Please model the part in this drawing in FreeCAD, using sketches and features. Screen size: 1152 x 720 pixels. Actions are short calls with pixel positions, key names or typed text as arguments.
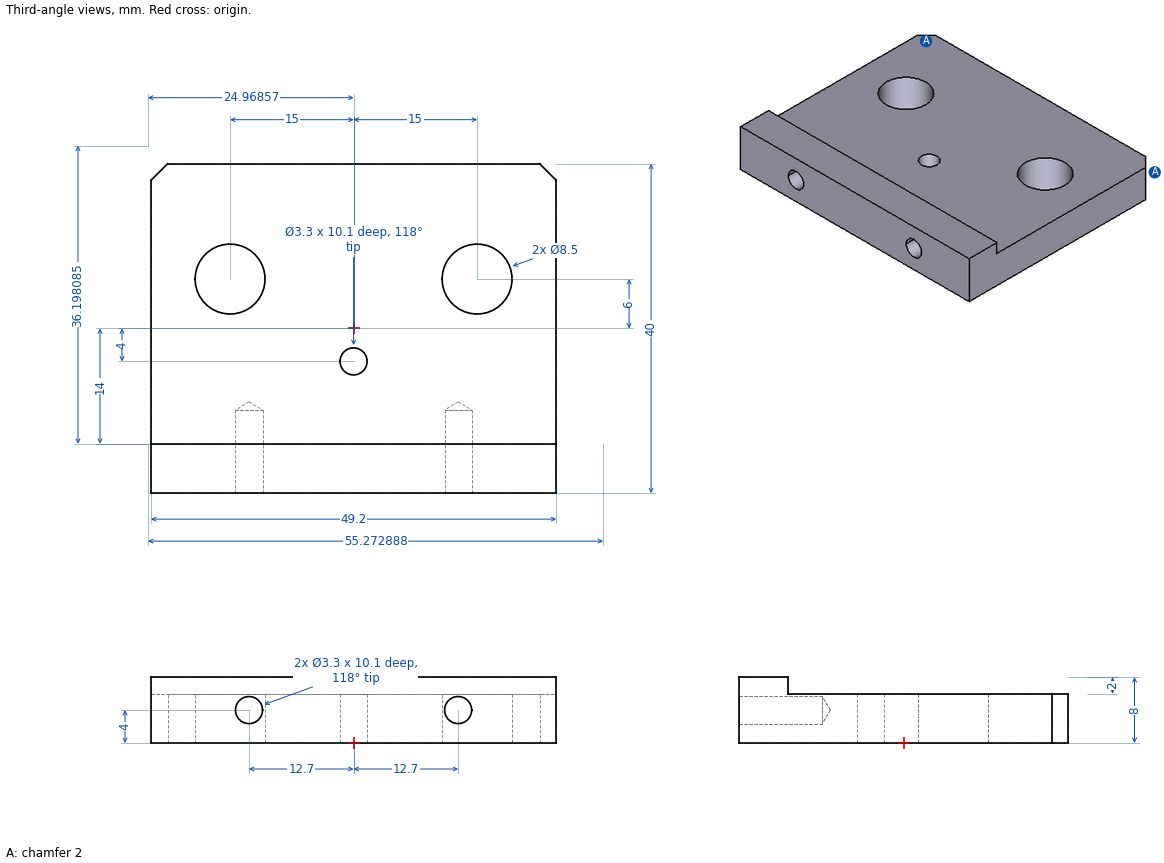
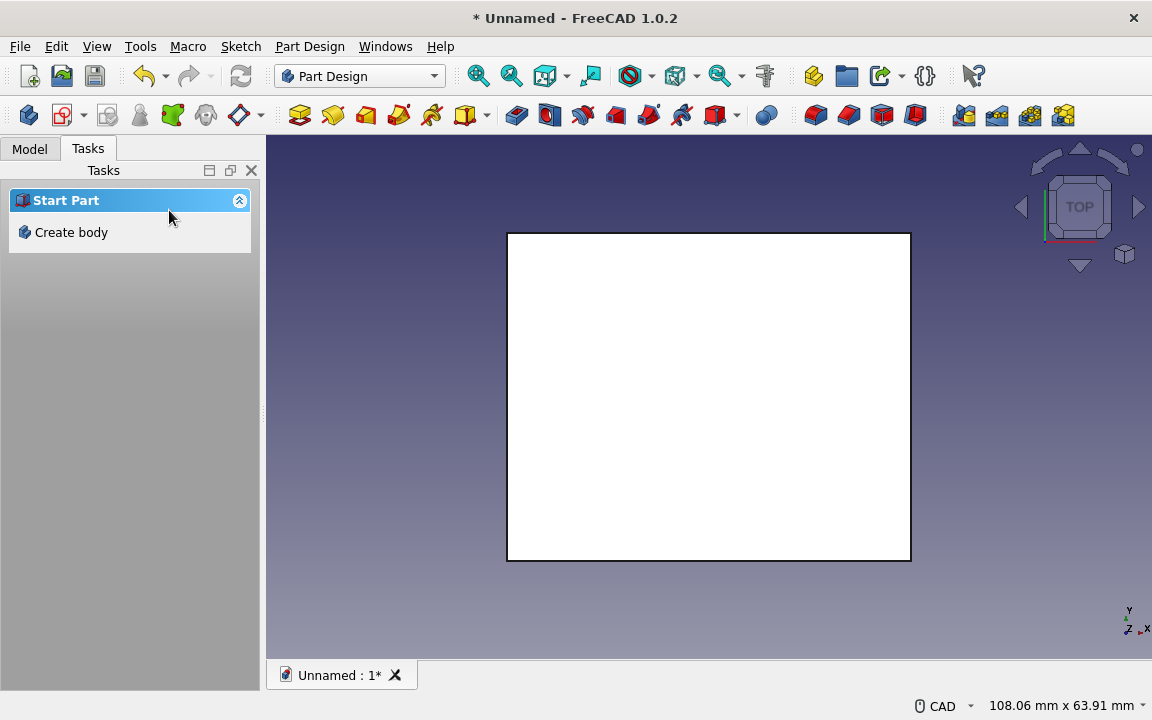
key(1)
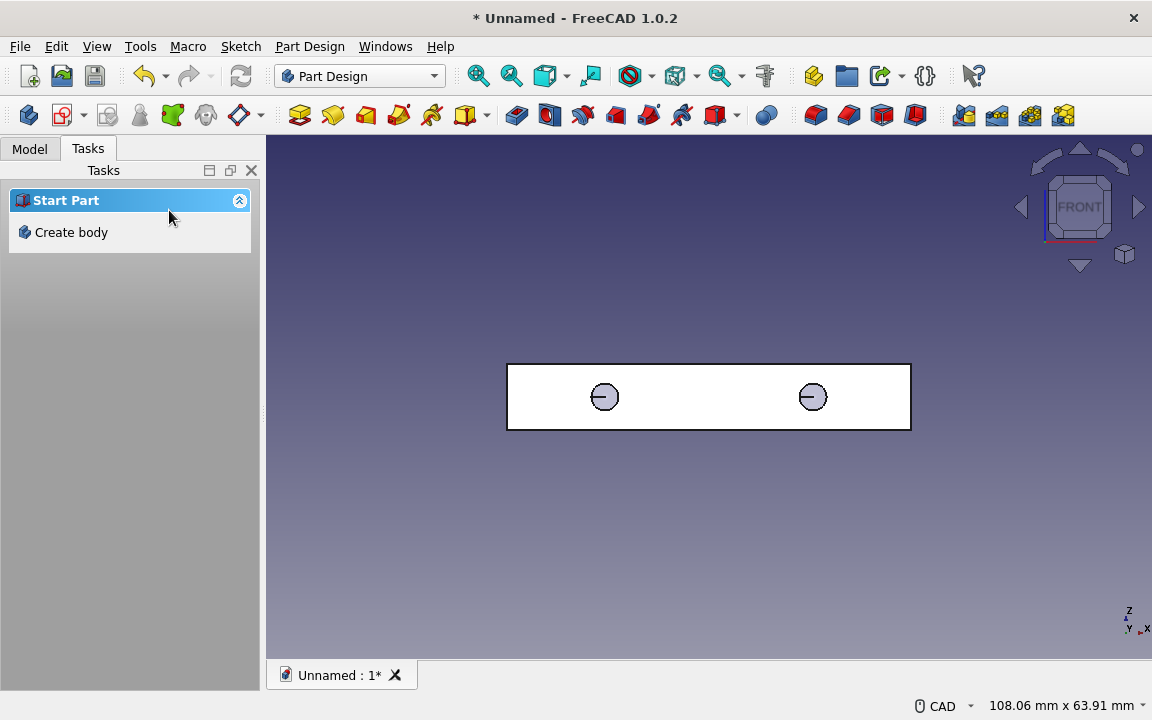
key(3)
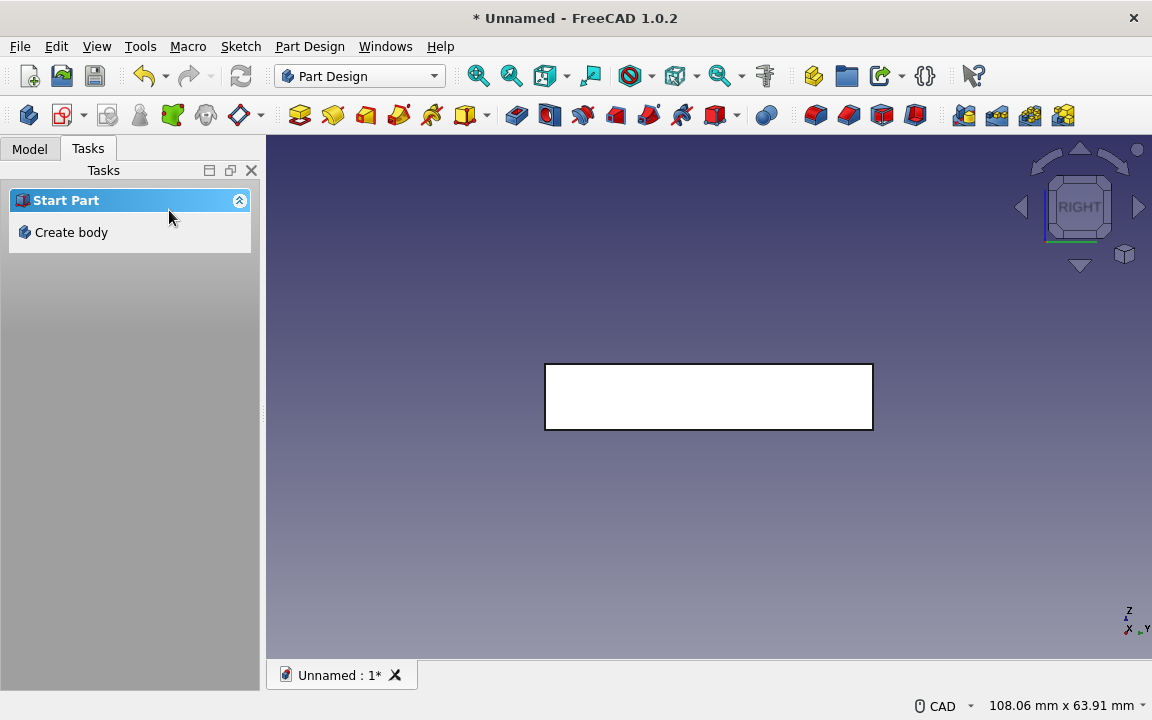
click(479, 76)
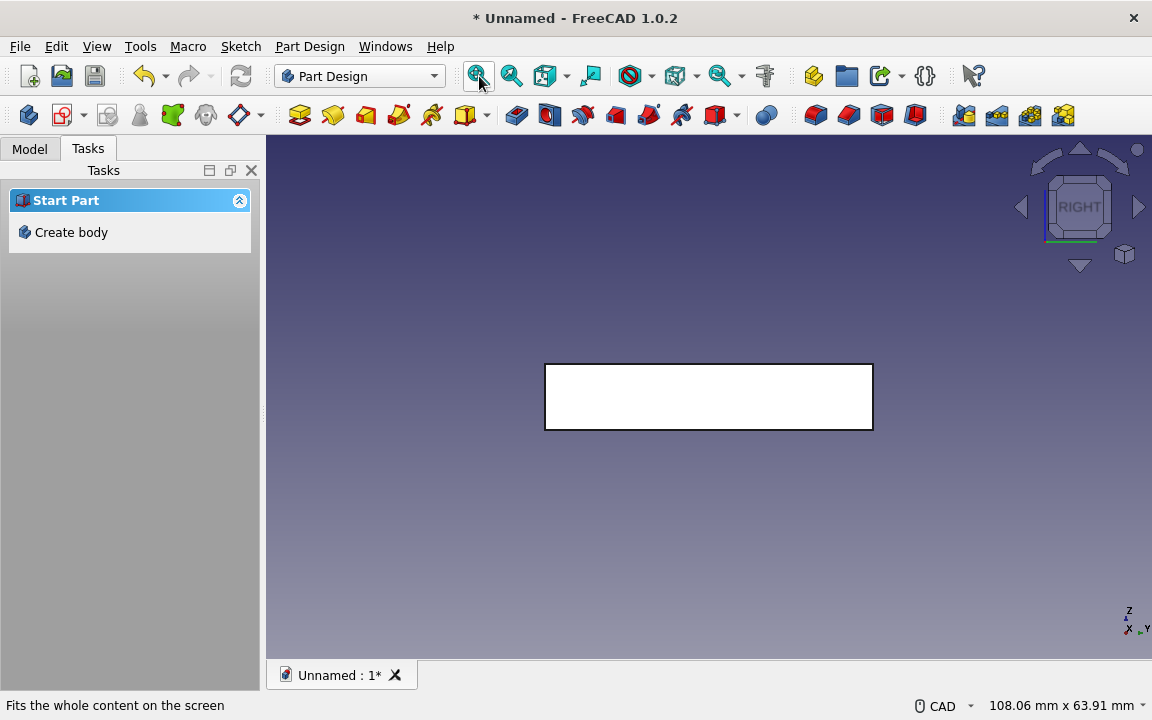
click(873, 396)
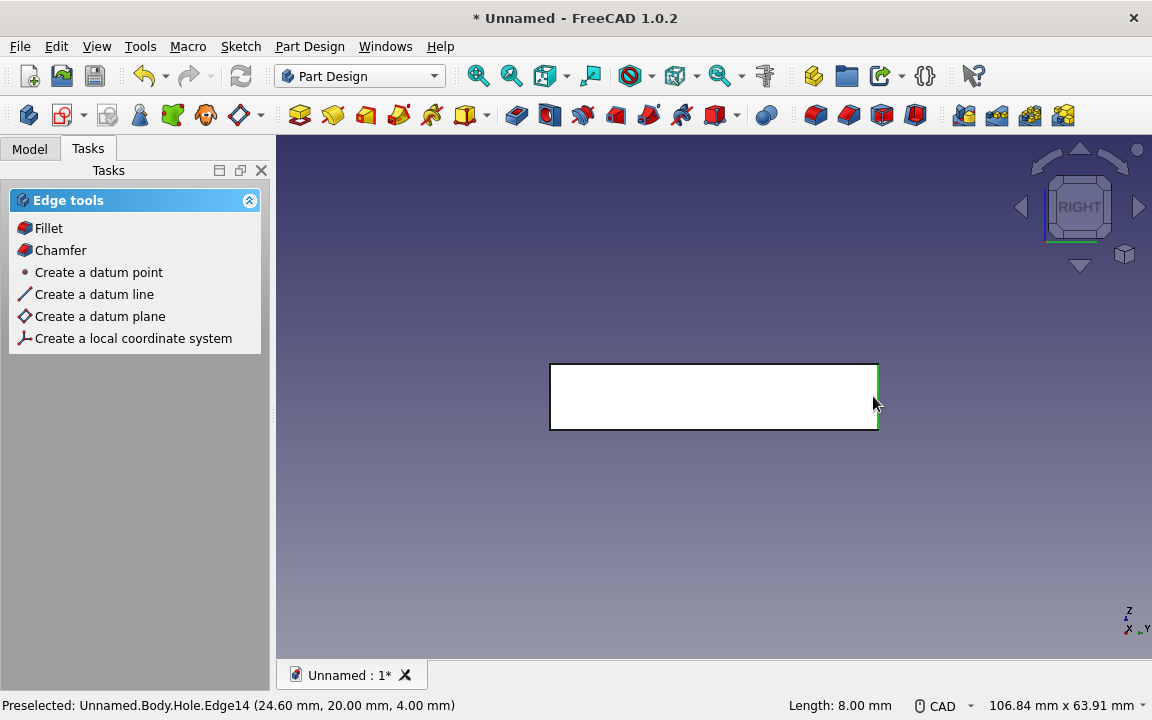
key(5)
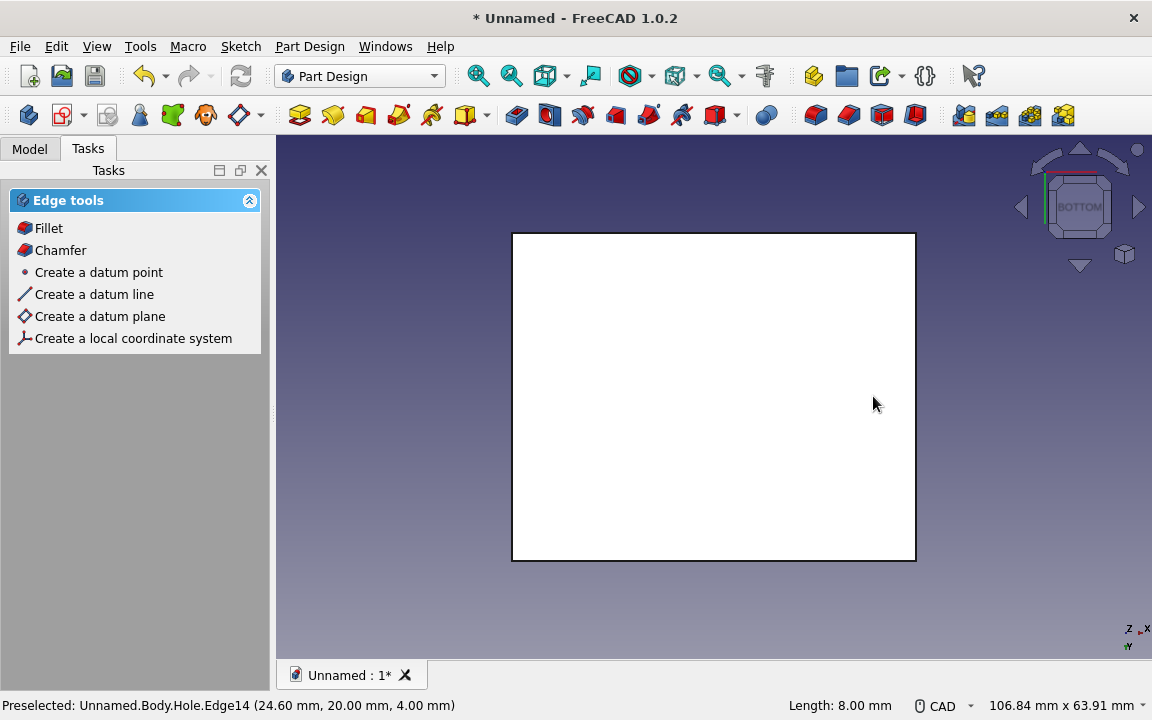
key(4)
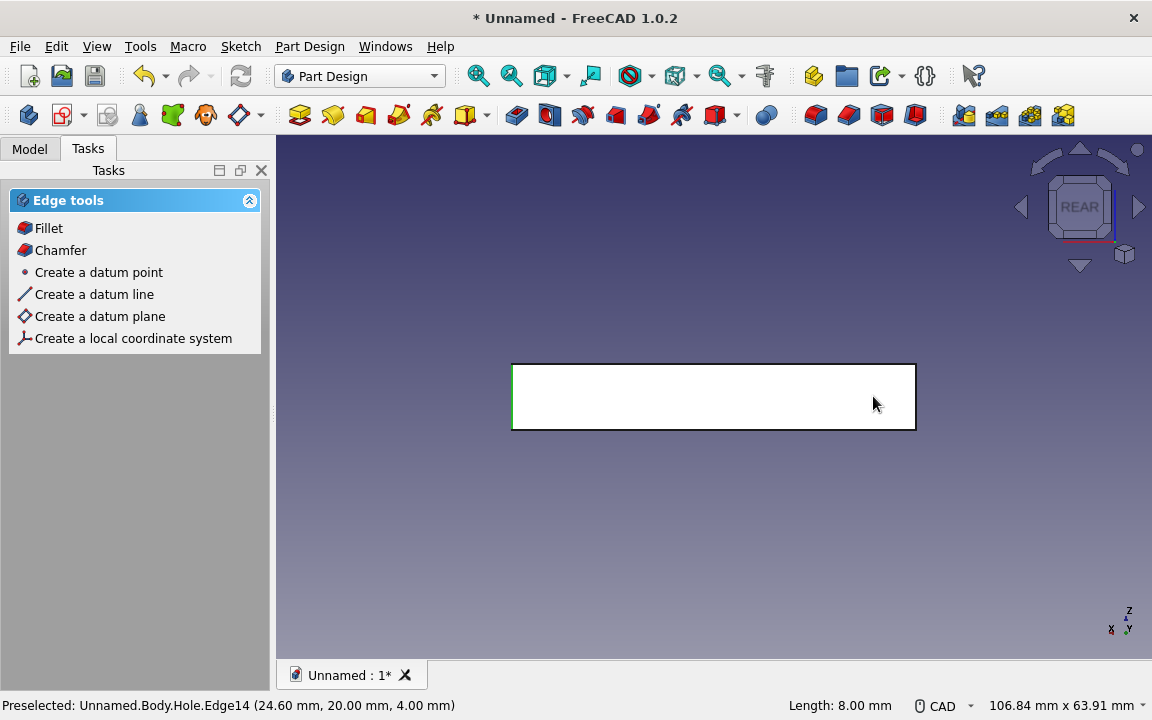
click(916, 396, ctrl)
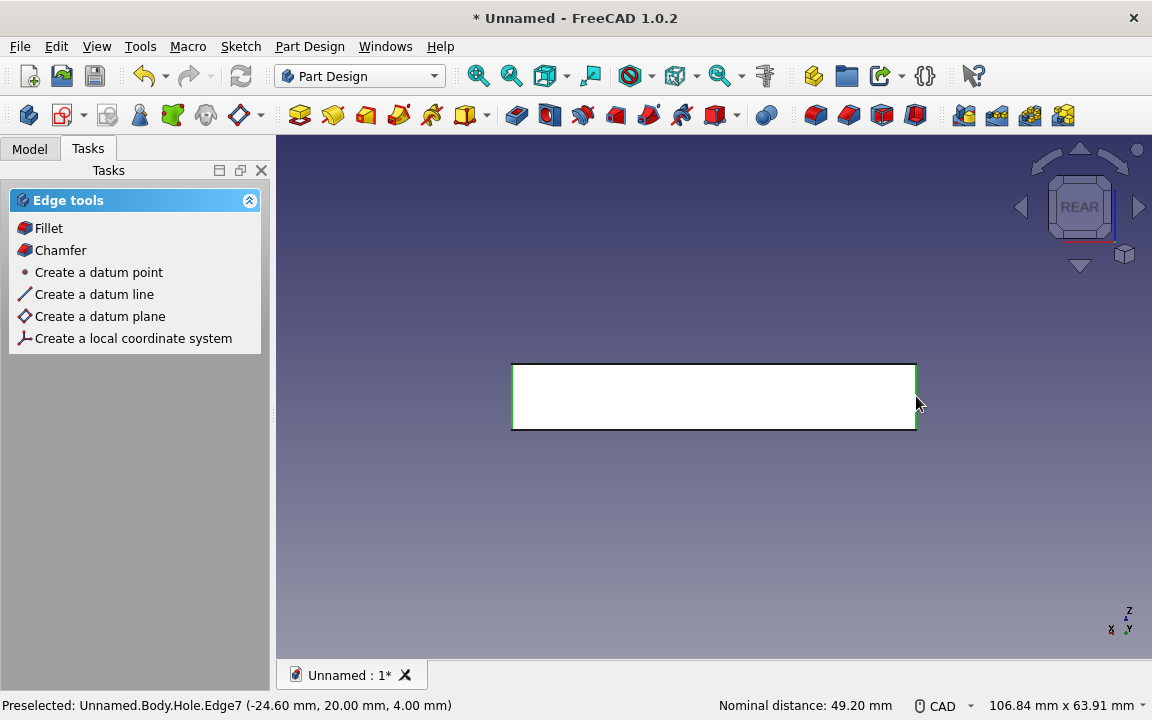
click(849, 116)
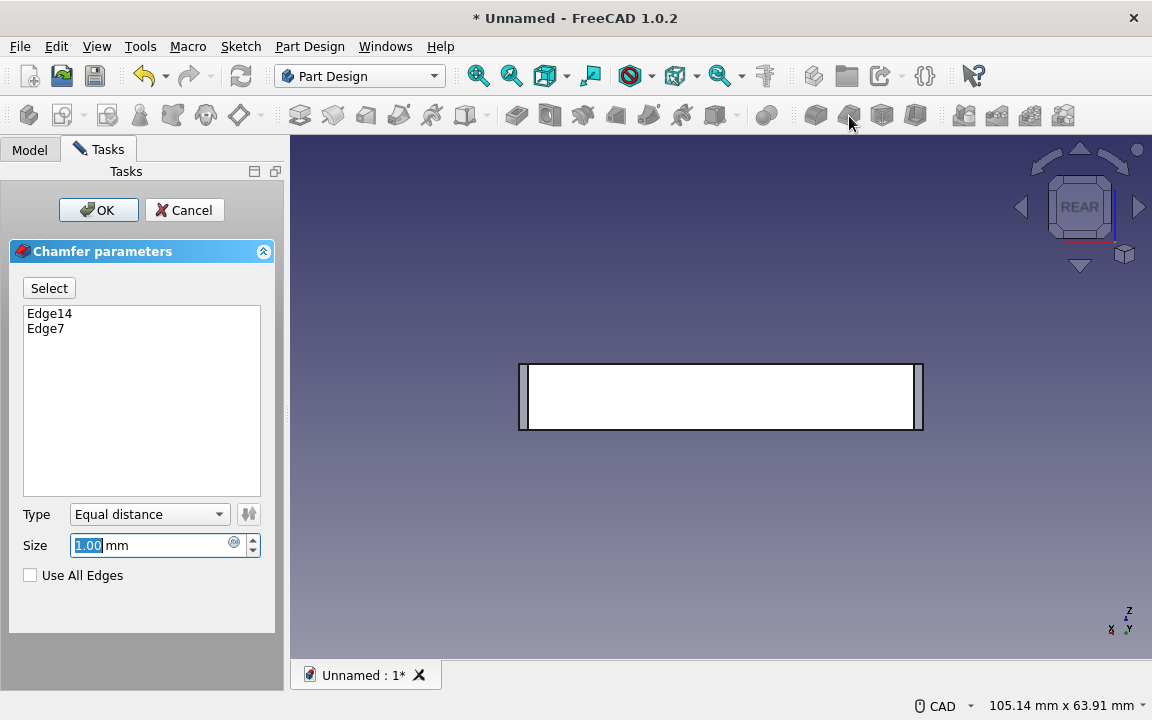
text(2)
key(Tab)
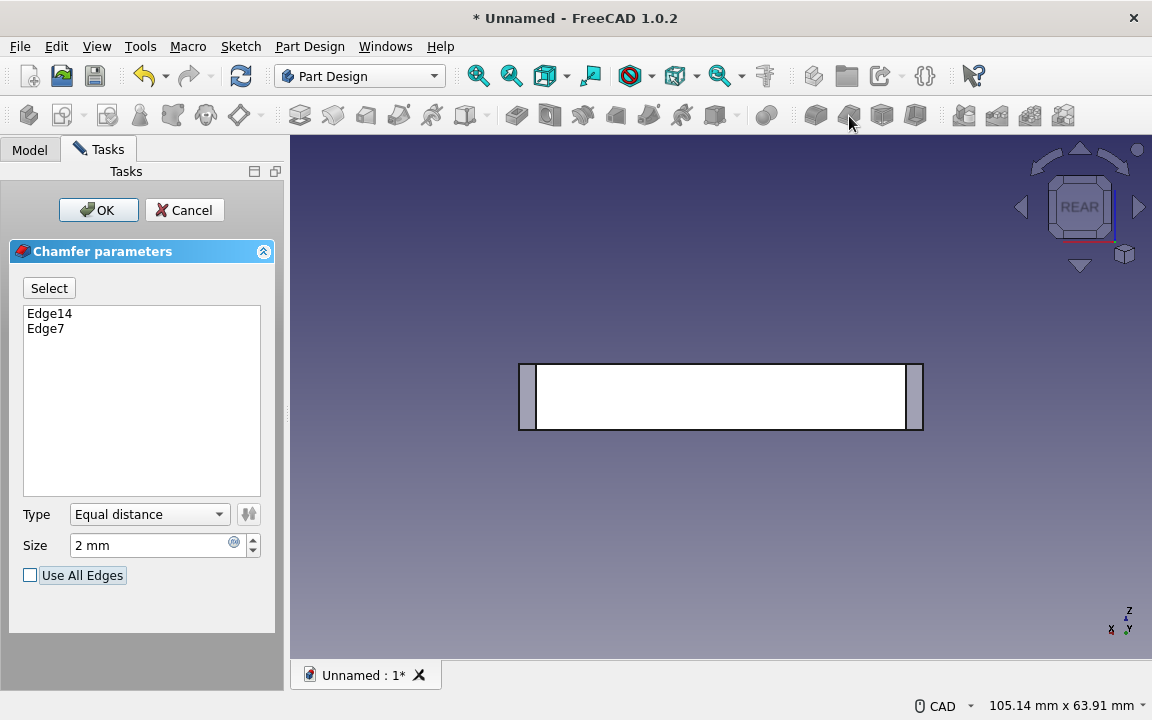
click(99, 210)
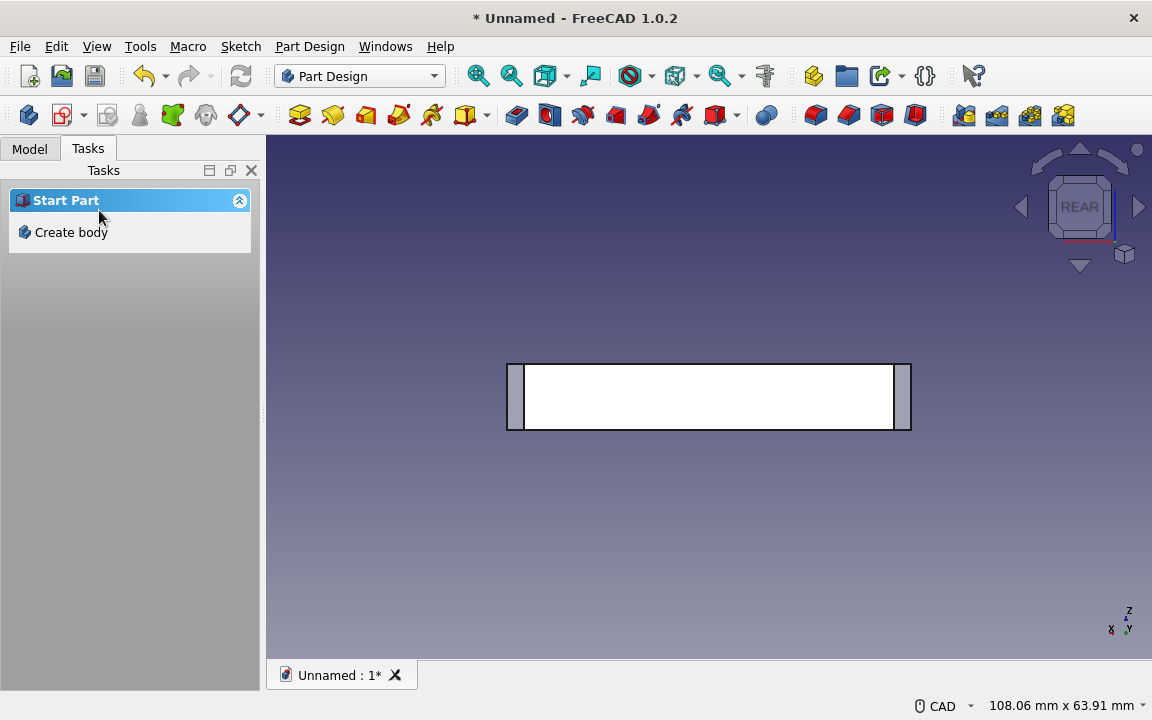
key(0)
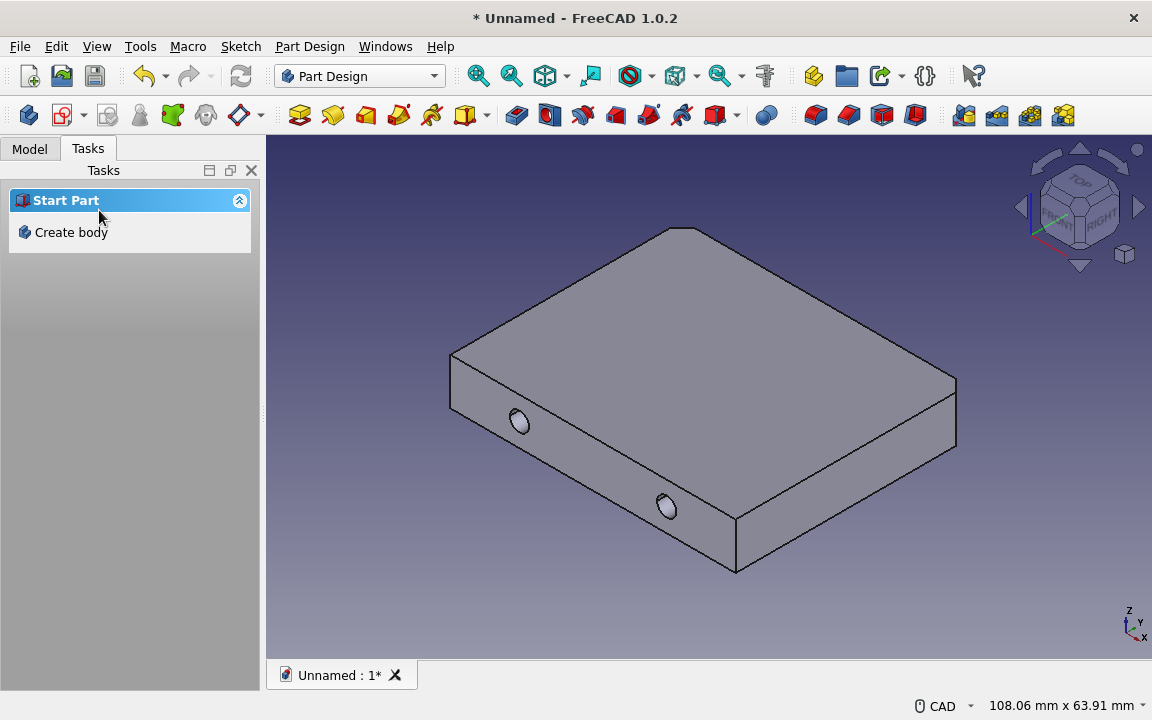
click(709, 369)